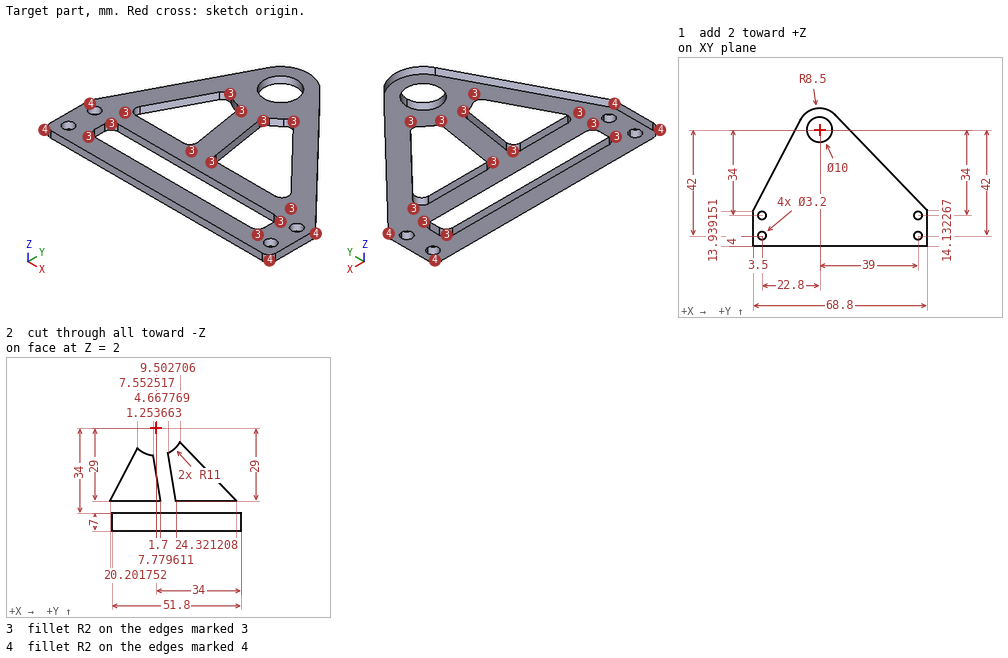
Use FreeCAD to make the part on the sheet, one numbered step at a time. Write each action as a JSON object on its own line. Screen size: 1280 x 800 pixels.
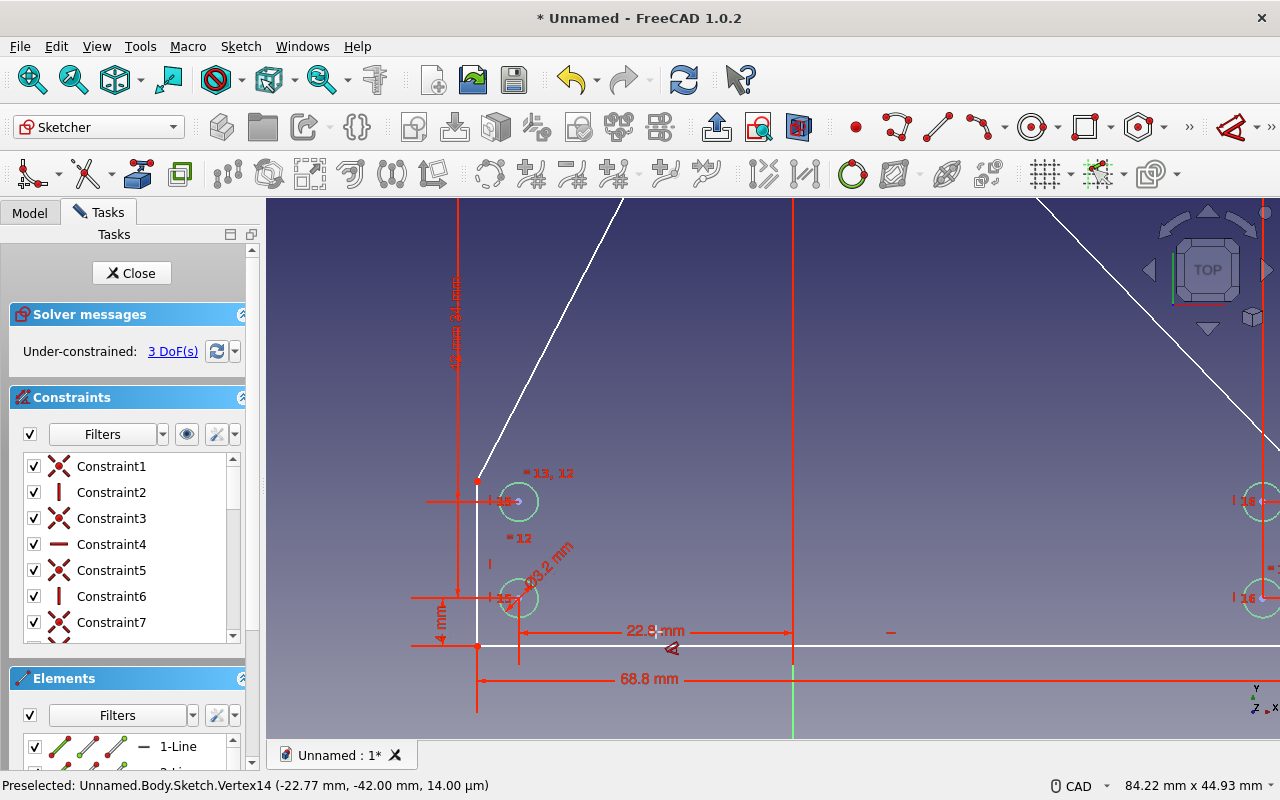
{"action": "left_click", "coordinate": [477, 646]}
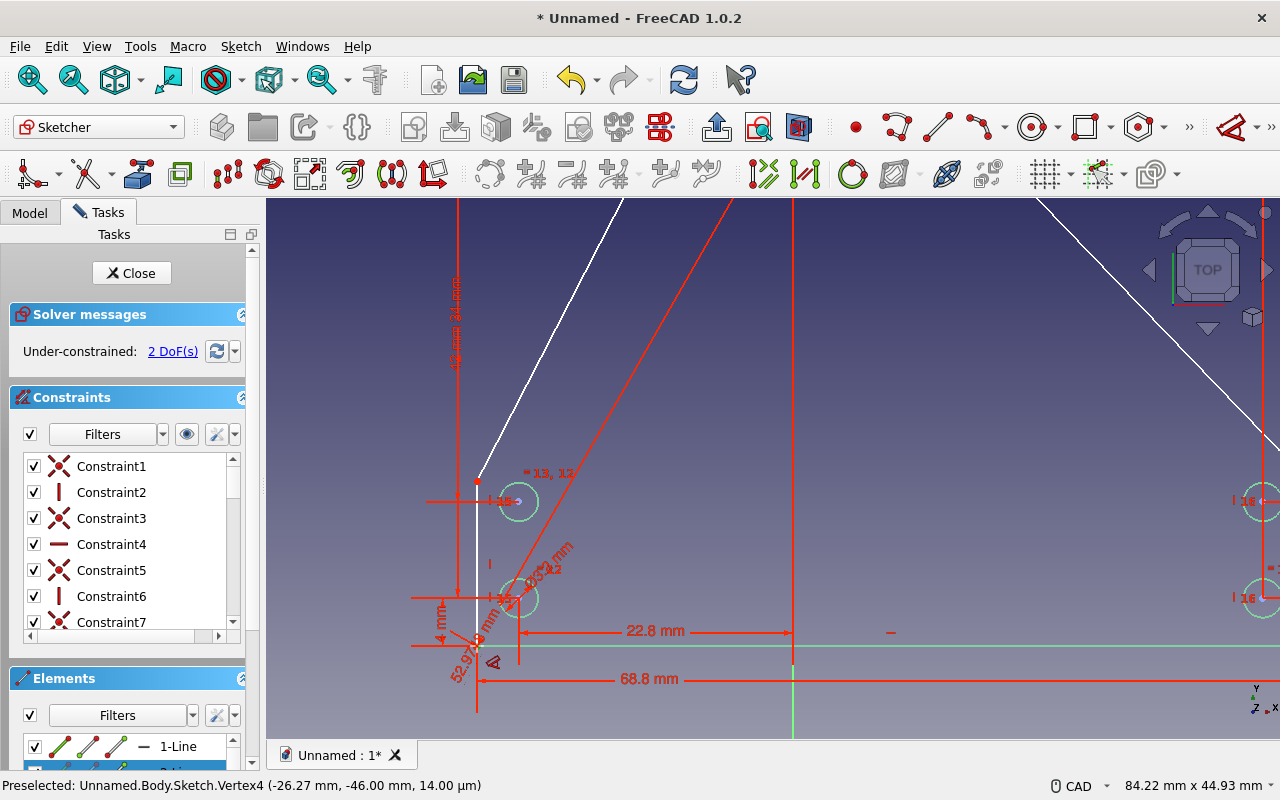
{"action": "left_click", "coordinate": [519, 598]}
{"action": "left_click", "coordinate": [498, 680]}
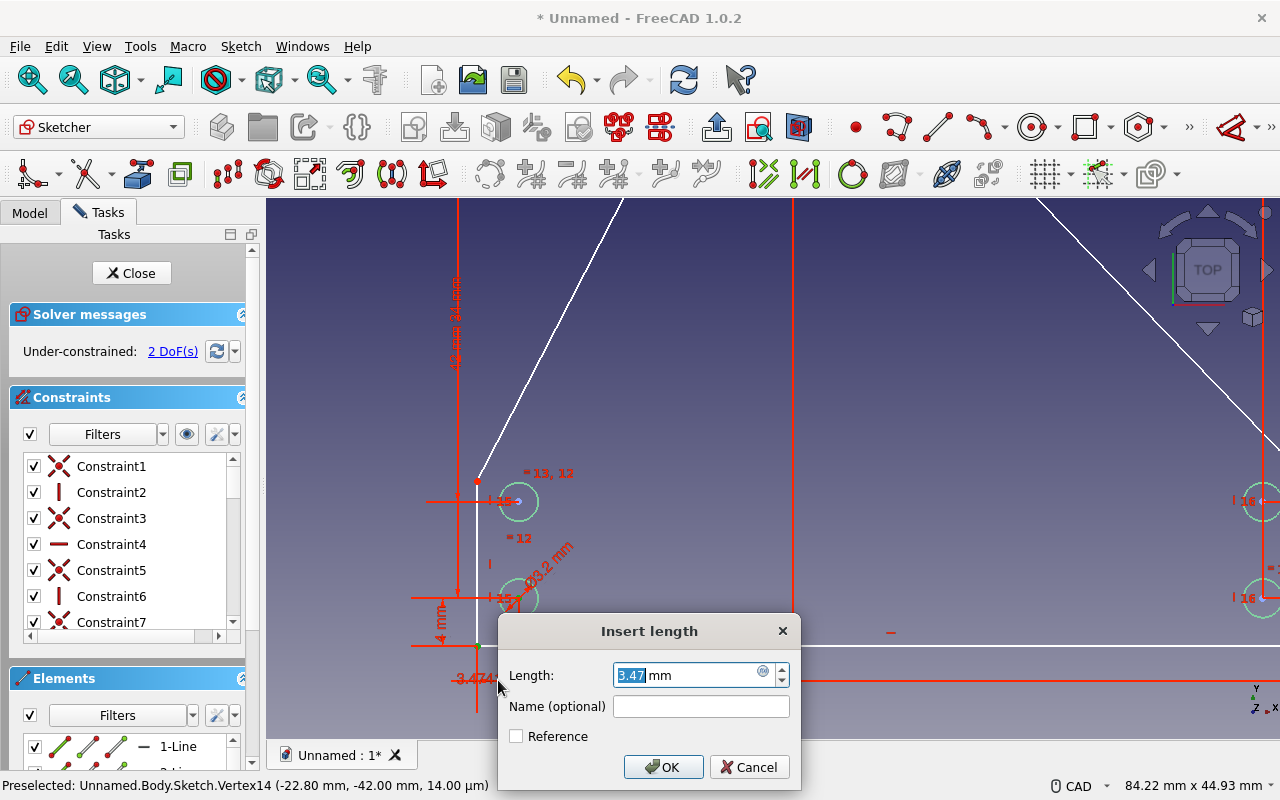
{"action": "type", "text": "3.5"}
{"action": "key", "text": "Return"}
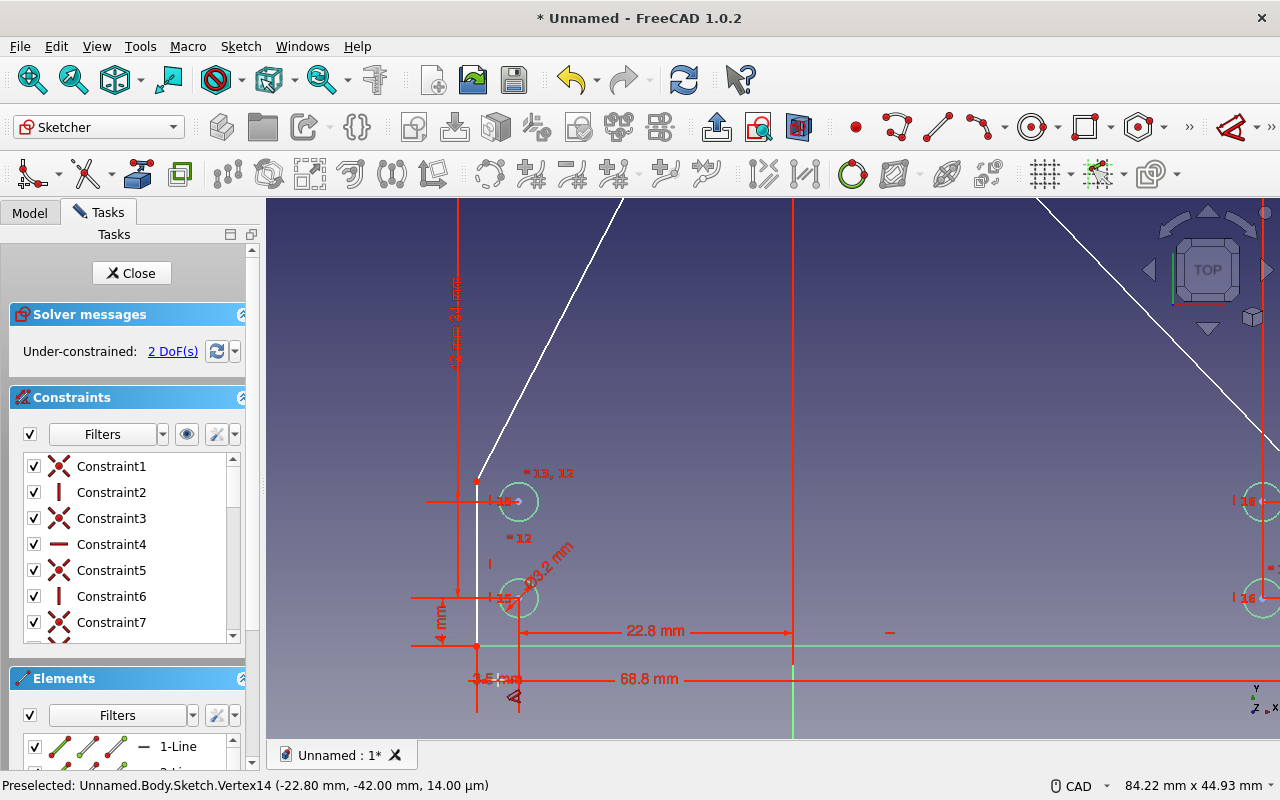
{"action": "left_click", "coordinate": [477, 531]}
{"action": "left_click", "coordinate": [443, 564]}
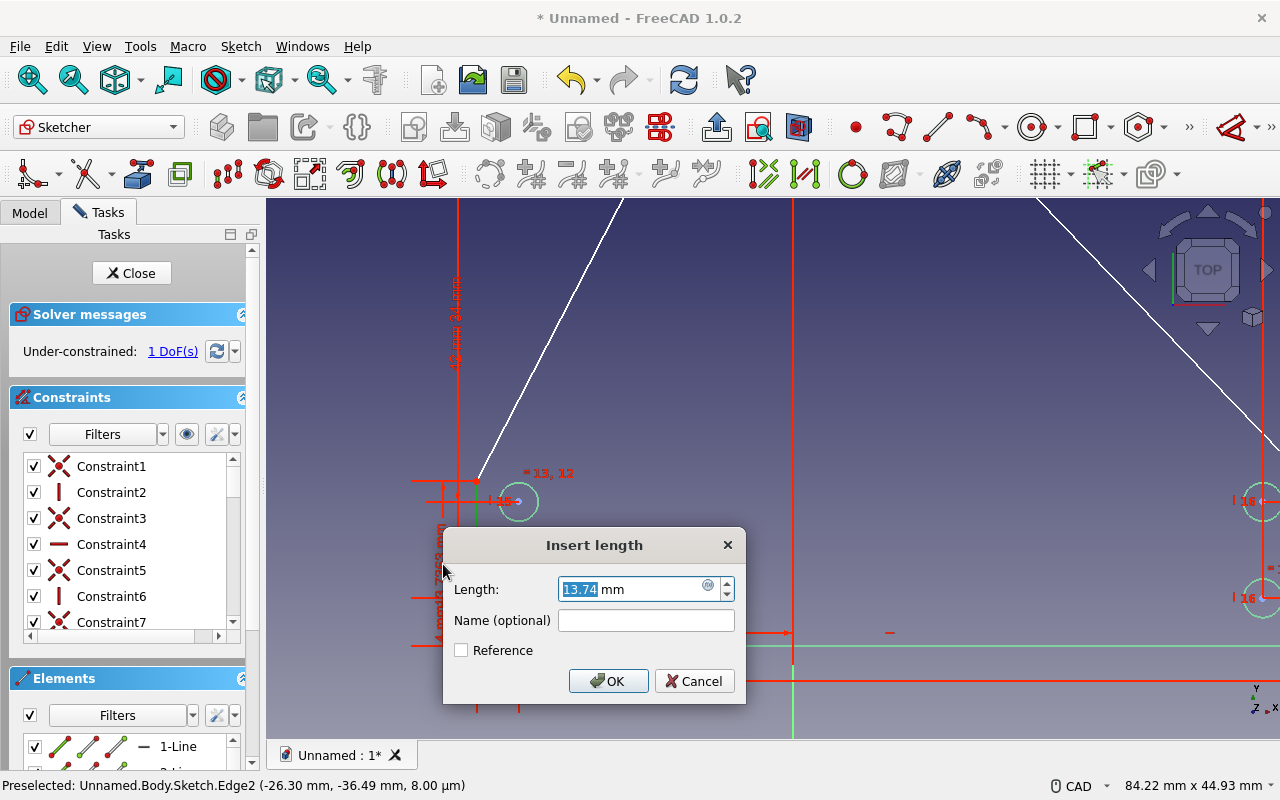
{"action": "type", "text": "13.939151"}
{"action": "key", "text": "Return"}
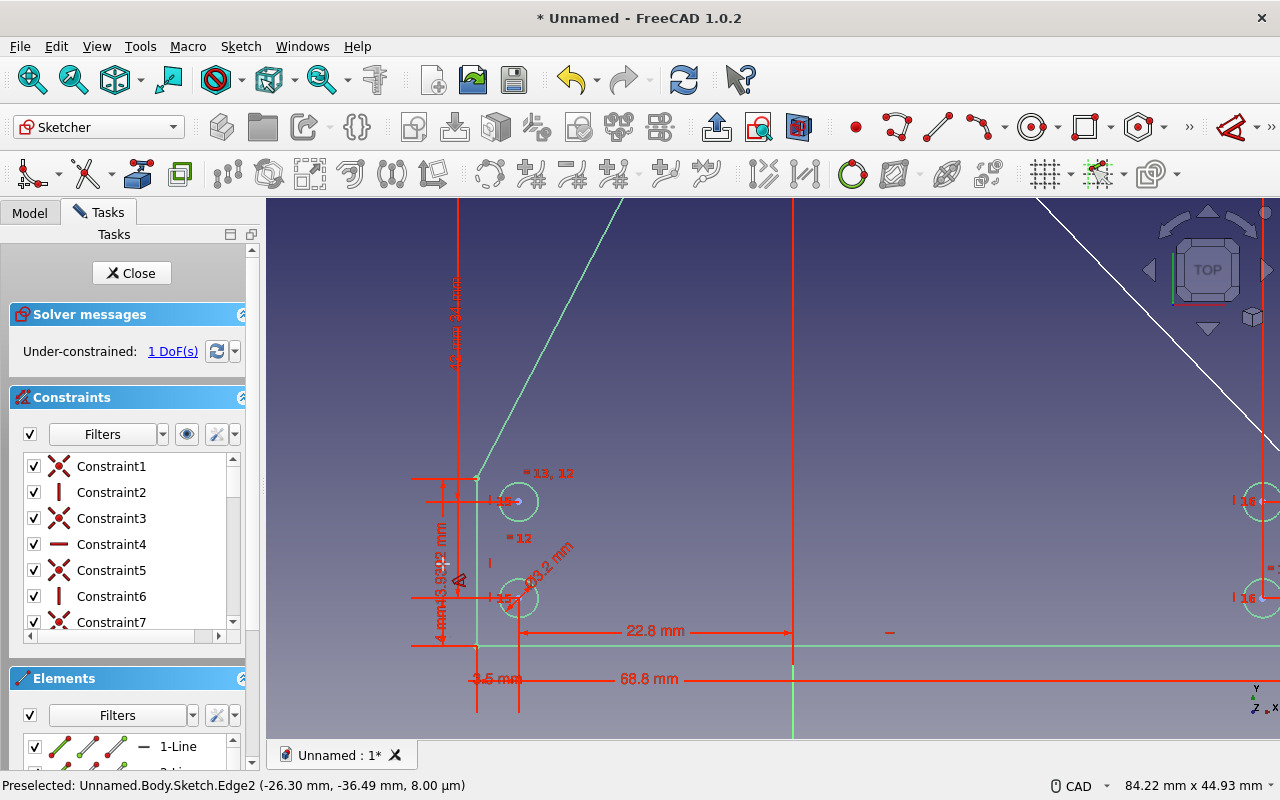
{"action": "scroll", "coordinate": [478, 650], "scroll_direction": "down", "scroll_amount": 3}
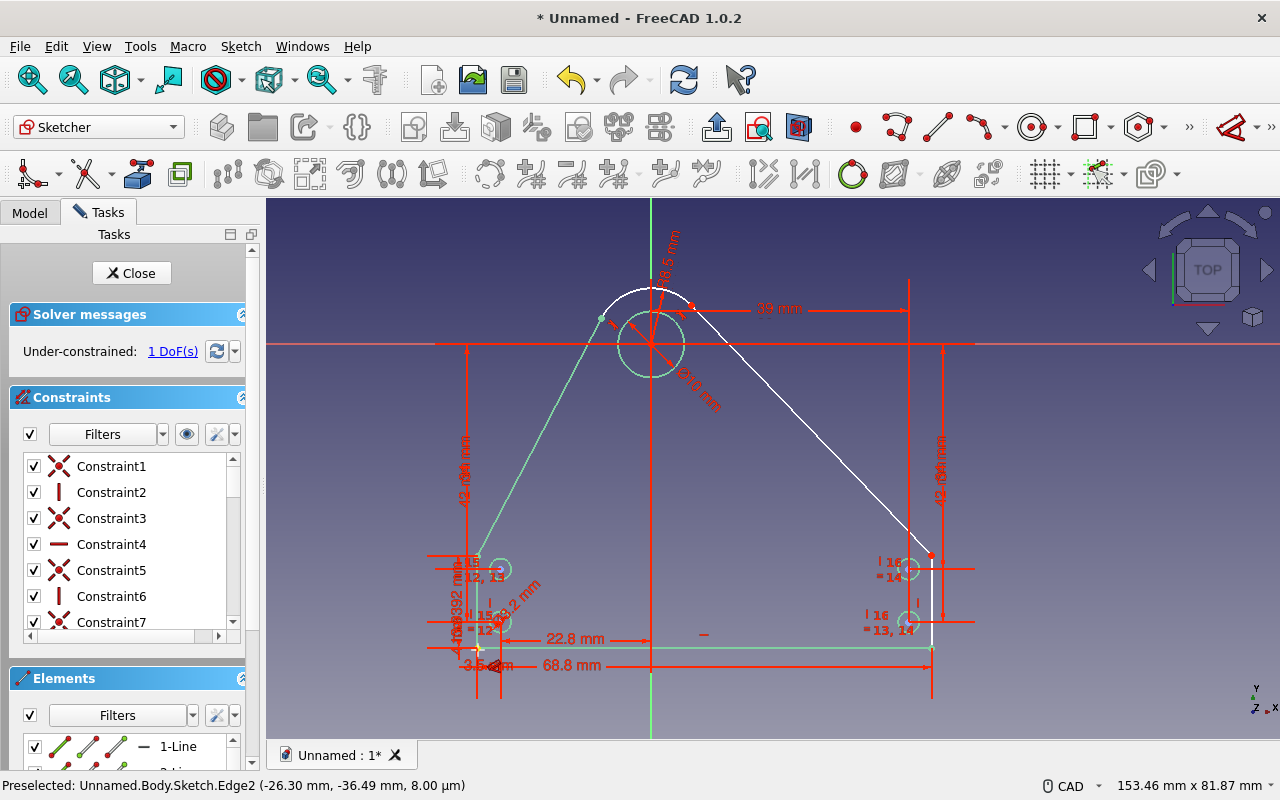
{"action": "left_click", "coordinate": [932, 621]}
{"action": "left_click", "coordinate": [966, 602]}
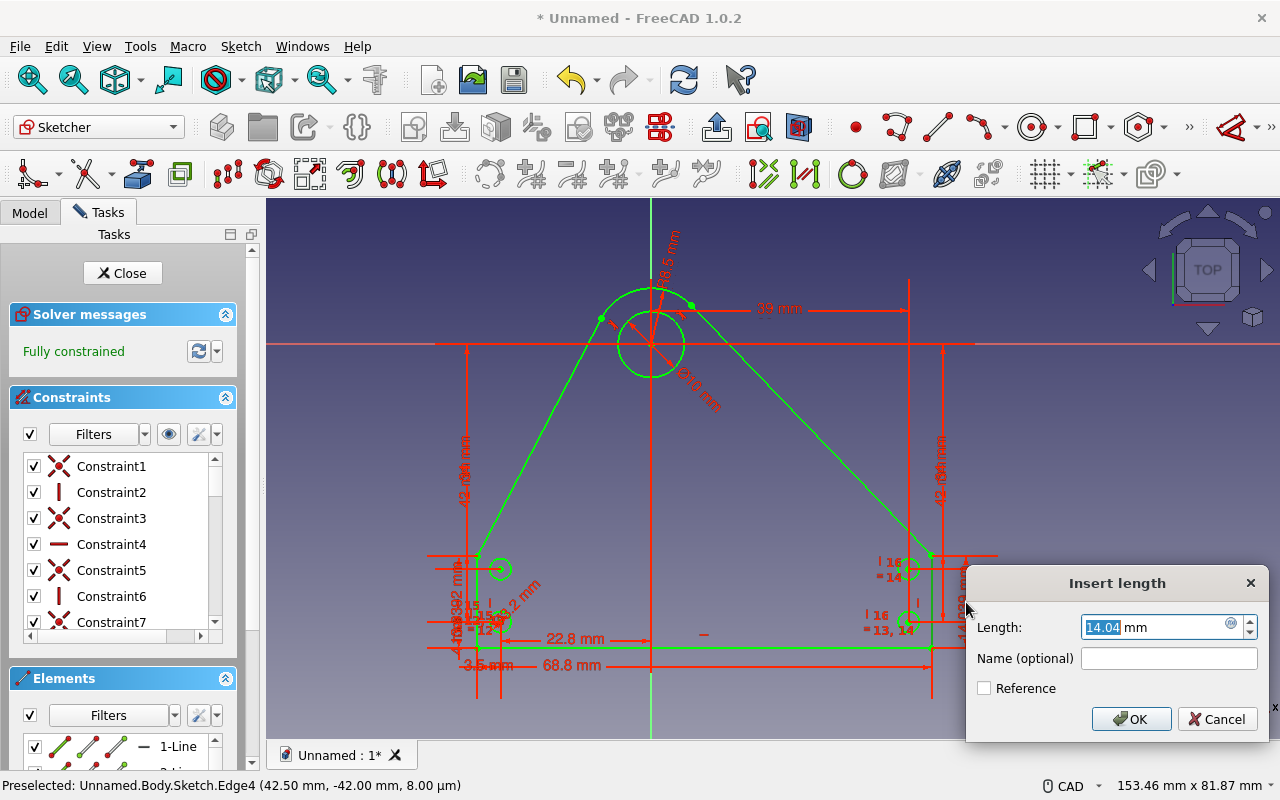
{"action": "type", "text": "14.132267"}
{"action": "key", "text": "Return"}
{"action": "key", "text": "Escape"}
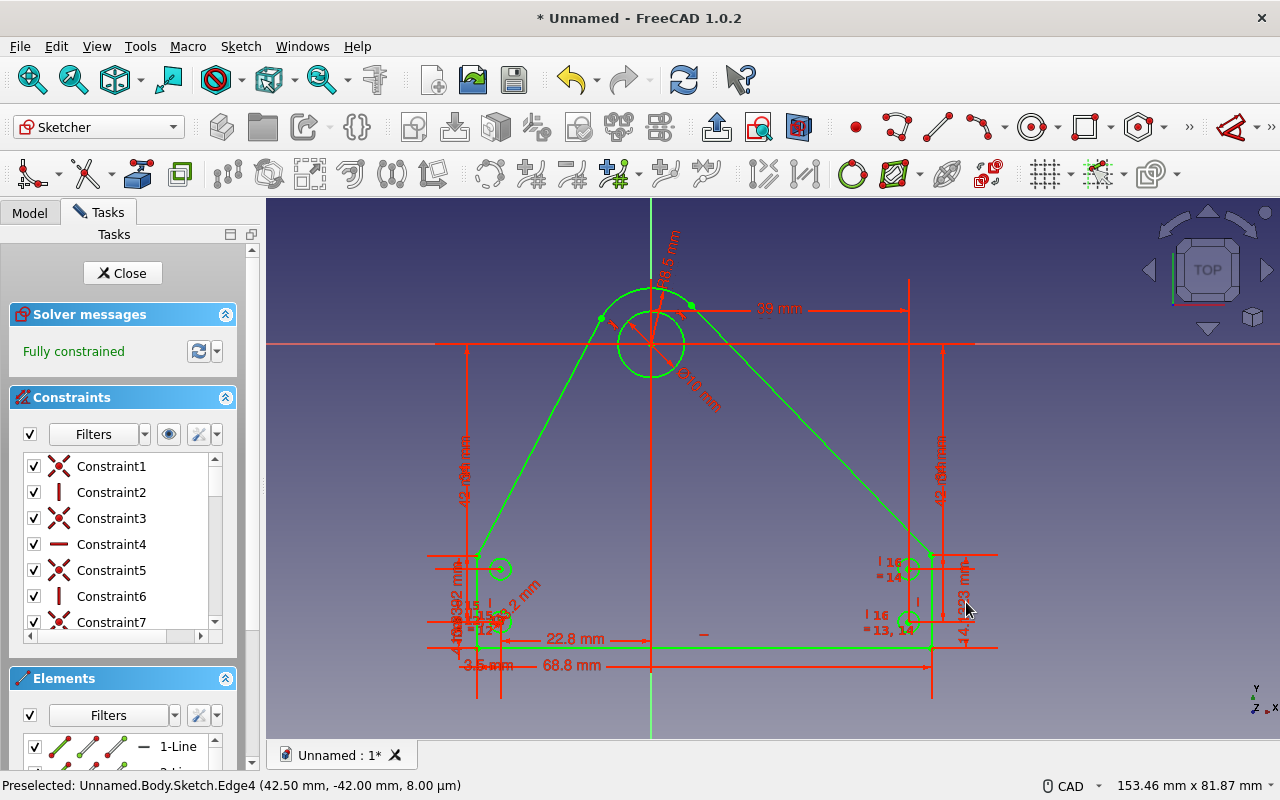
{"action": "left_click", "coordinate": [123, 273]}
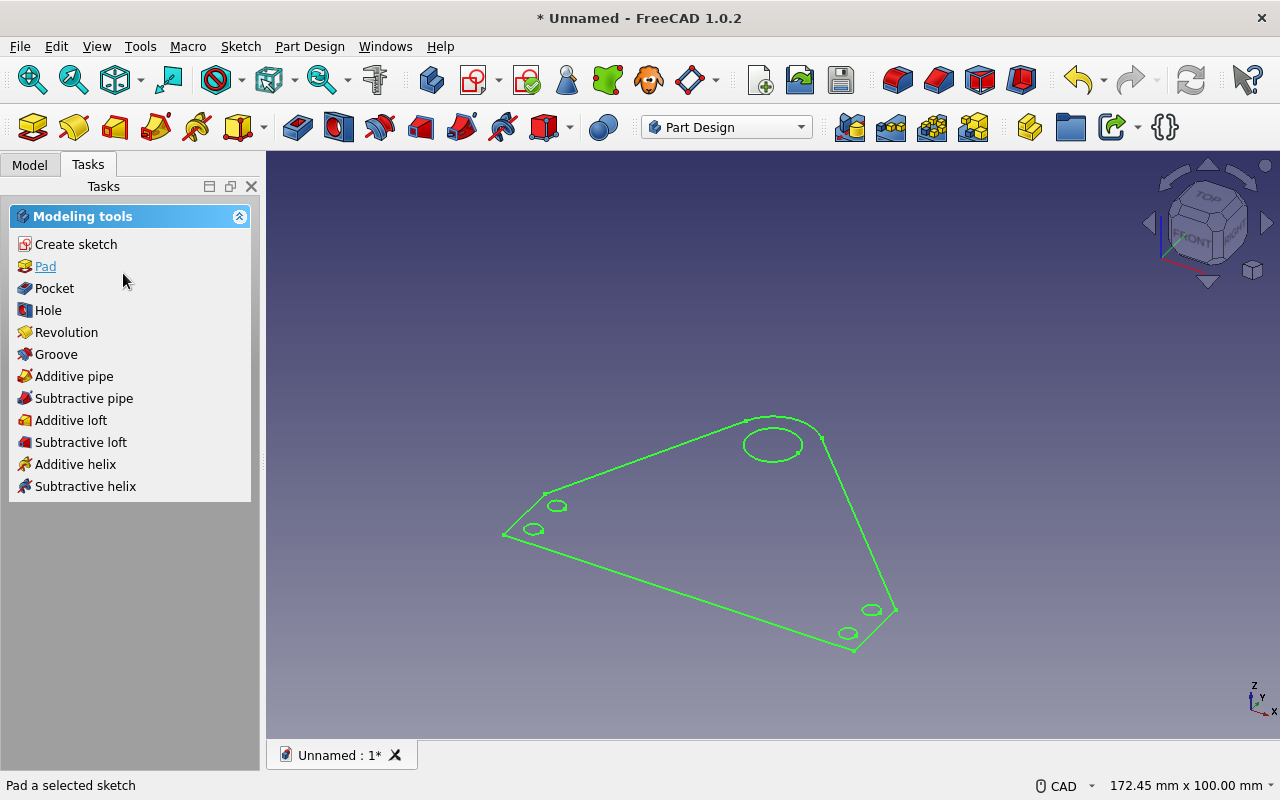
{"action": "left_click", "coordinate": [33, 128]}